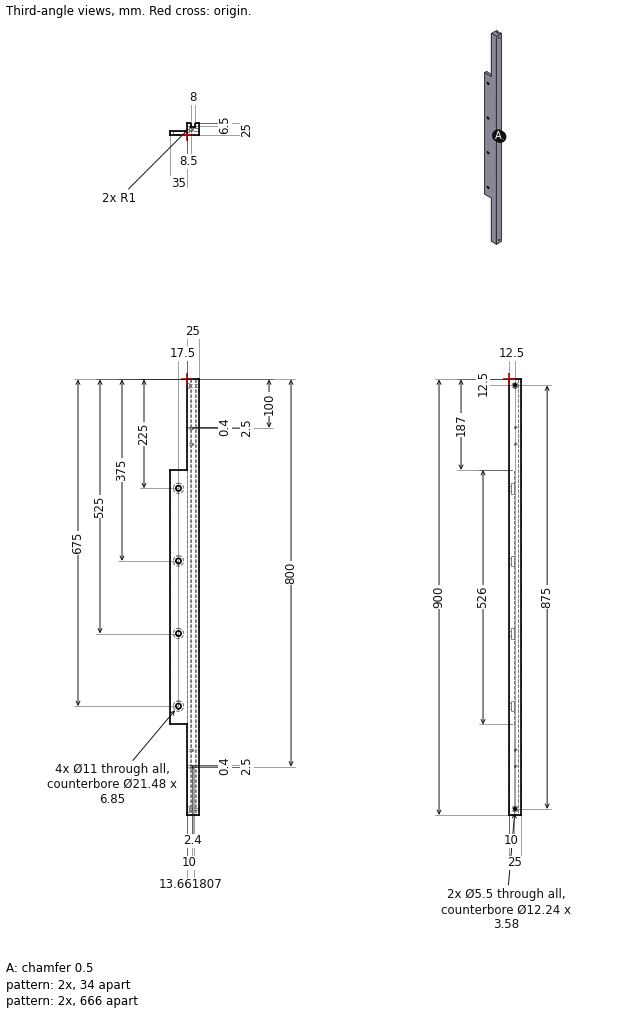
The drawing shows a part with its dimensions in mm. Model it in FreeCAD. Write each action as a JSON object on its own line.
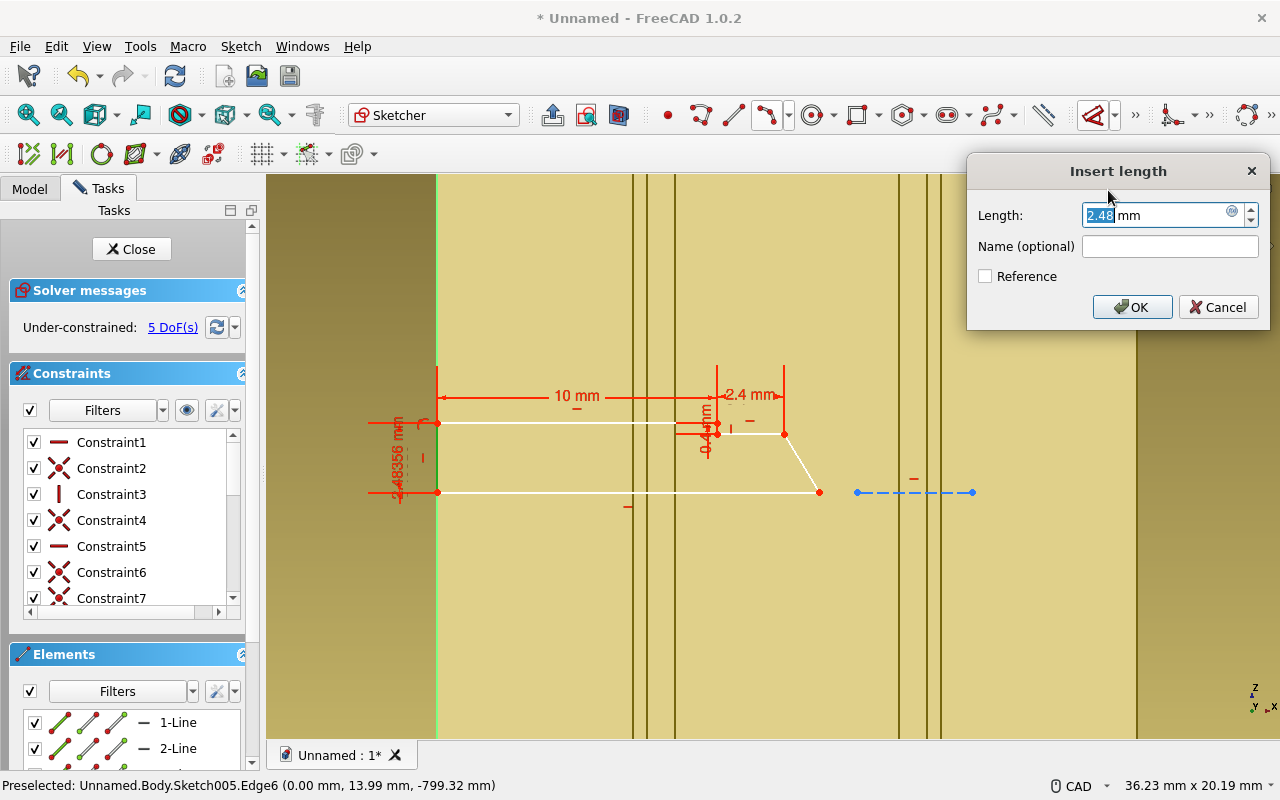
{"action": "type", "text": "2.5"}
{"action": "key", "text": "Return"}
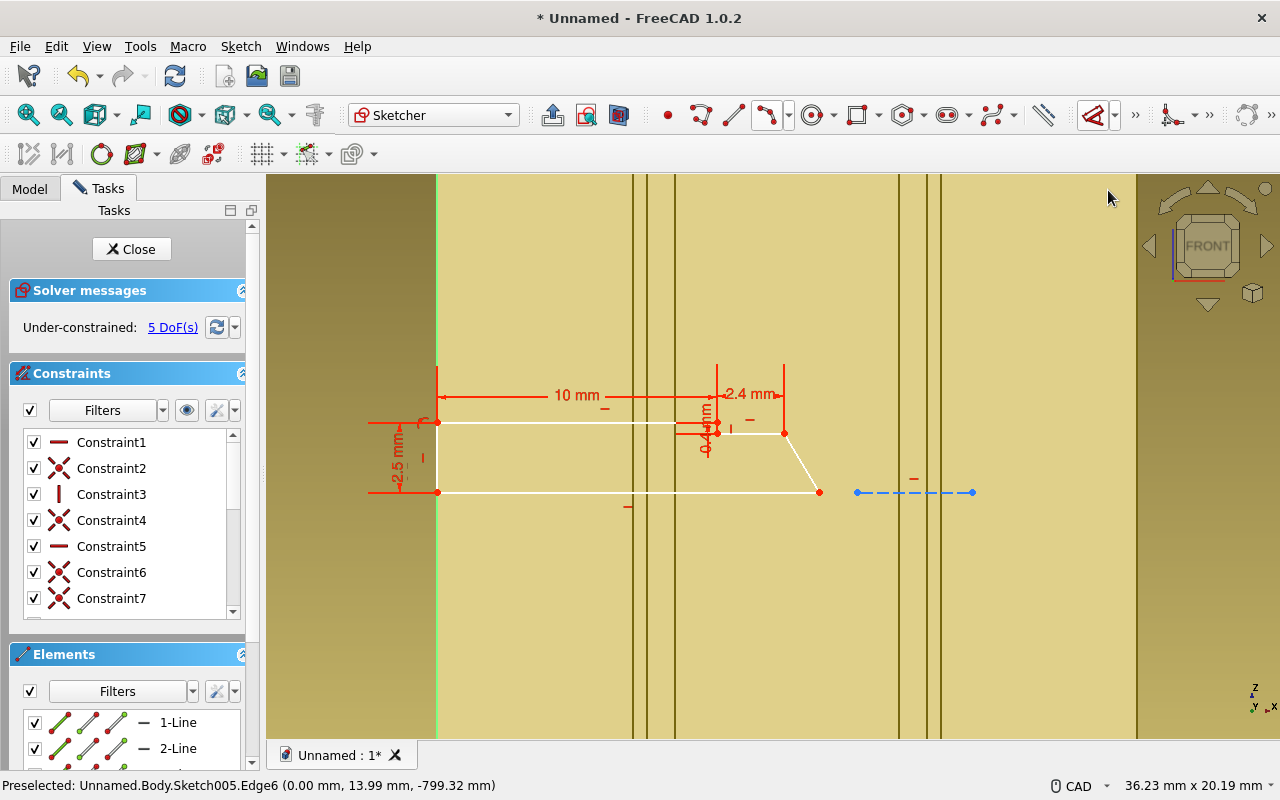
{"action": "left_click", "coordinate": [819, 493]}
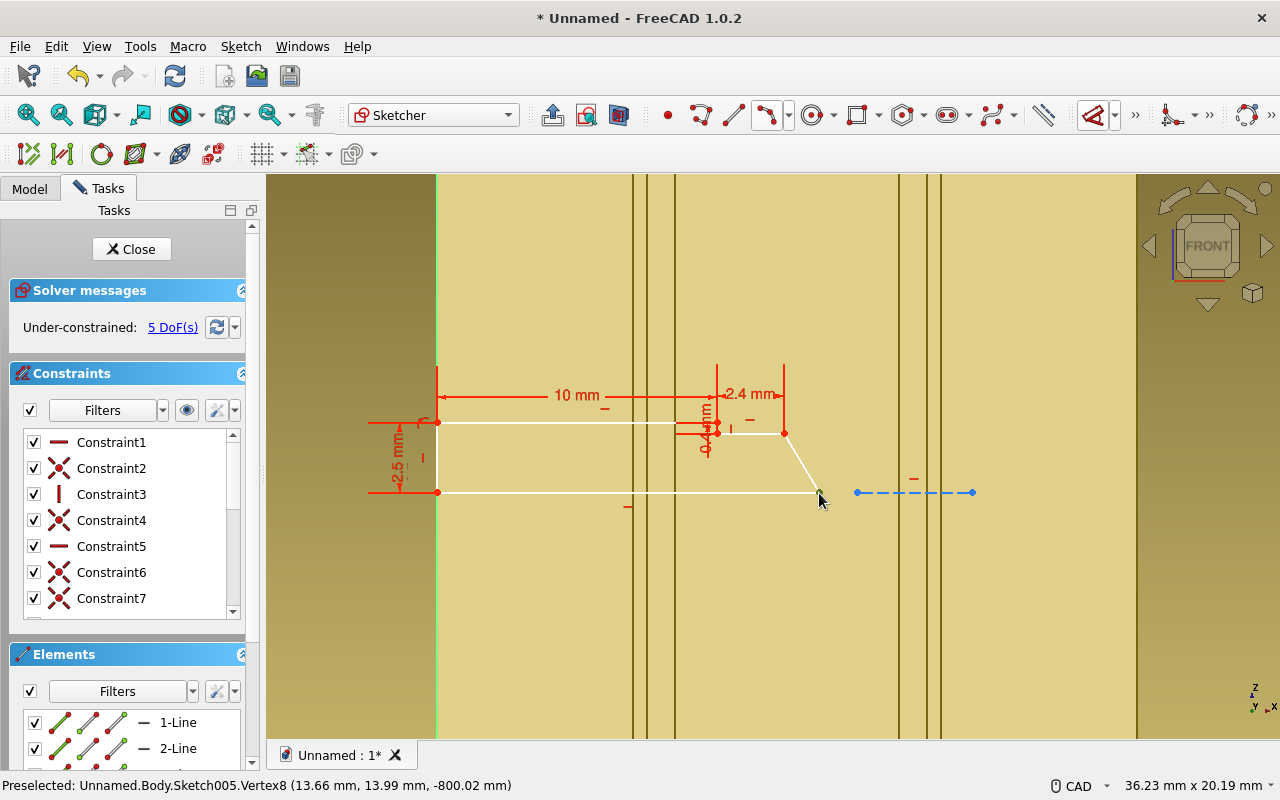
{"action": "left_click", "coordinate": [1114, 116]}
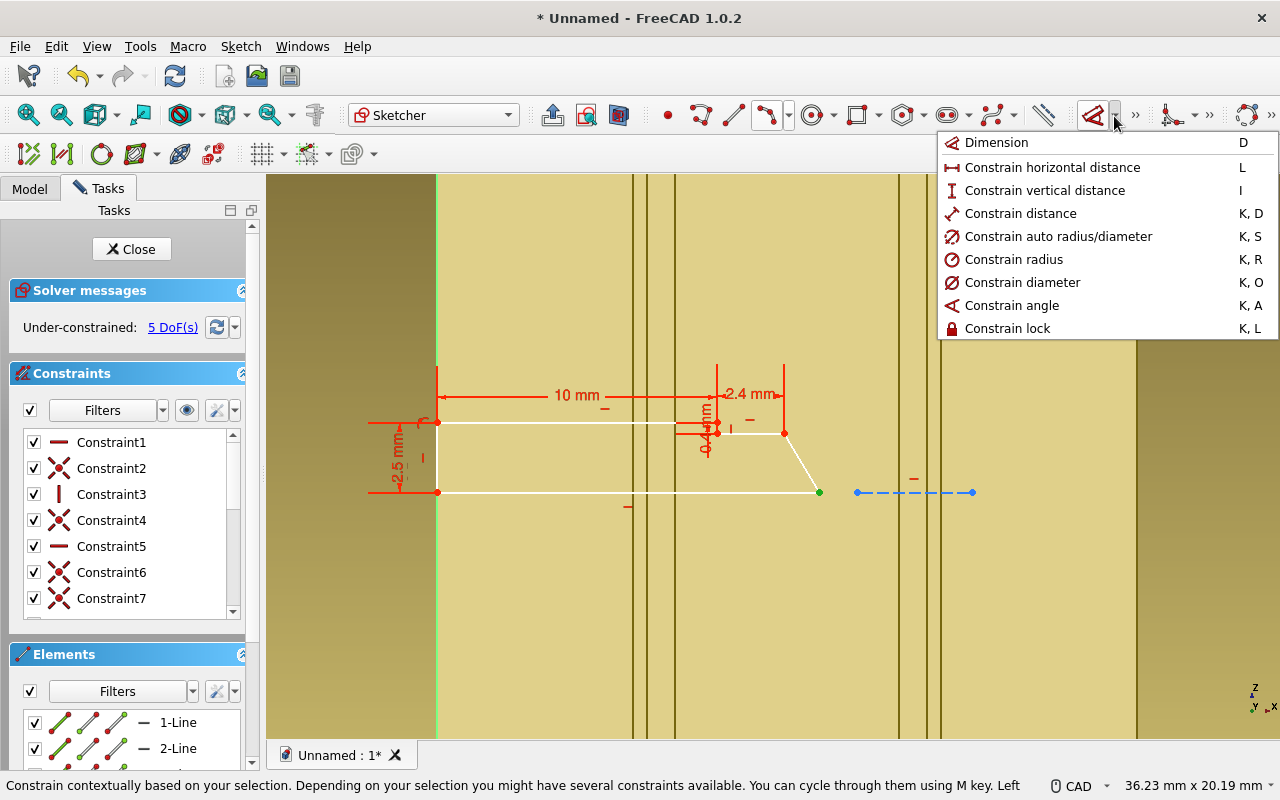
{"action": "left_click", "coordinate": [1108, 190]}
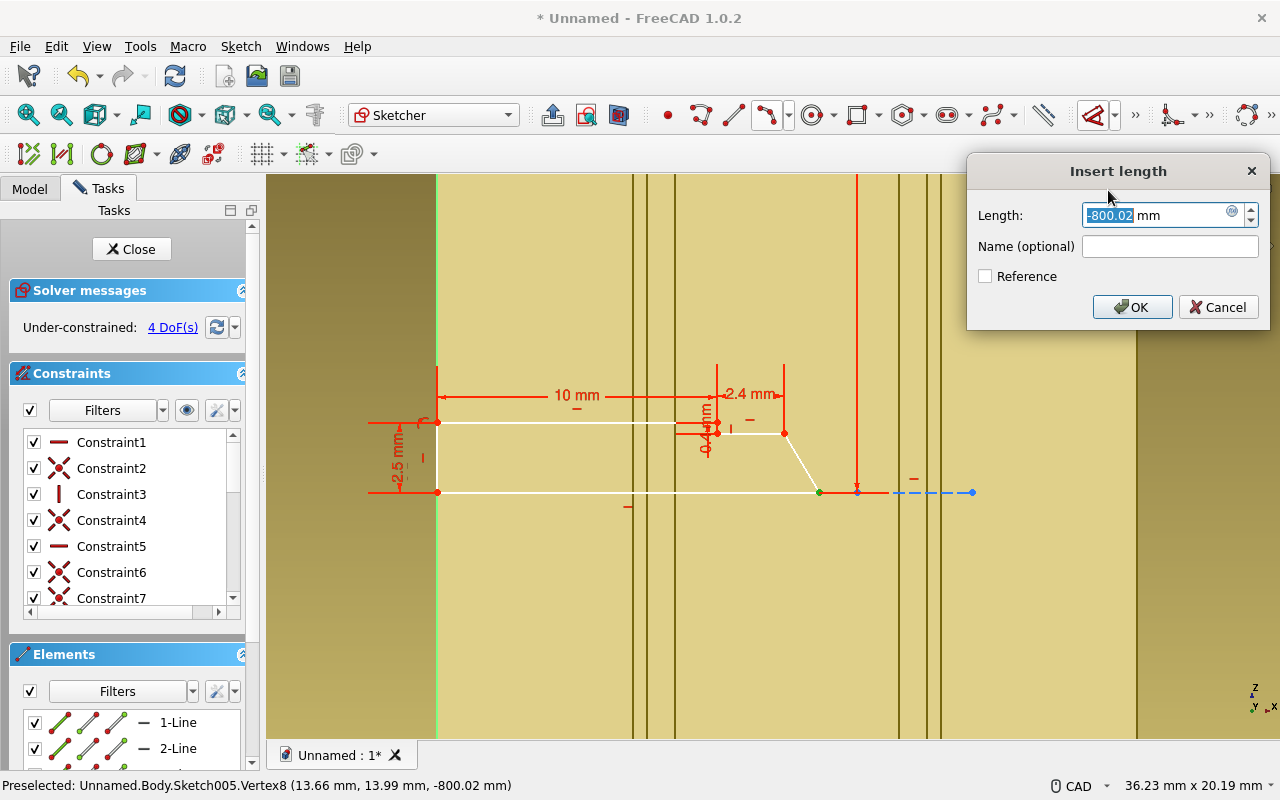
{"action": "type", "text": "-800"}
{"action": "key", "text": "Return"}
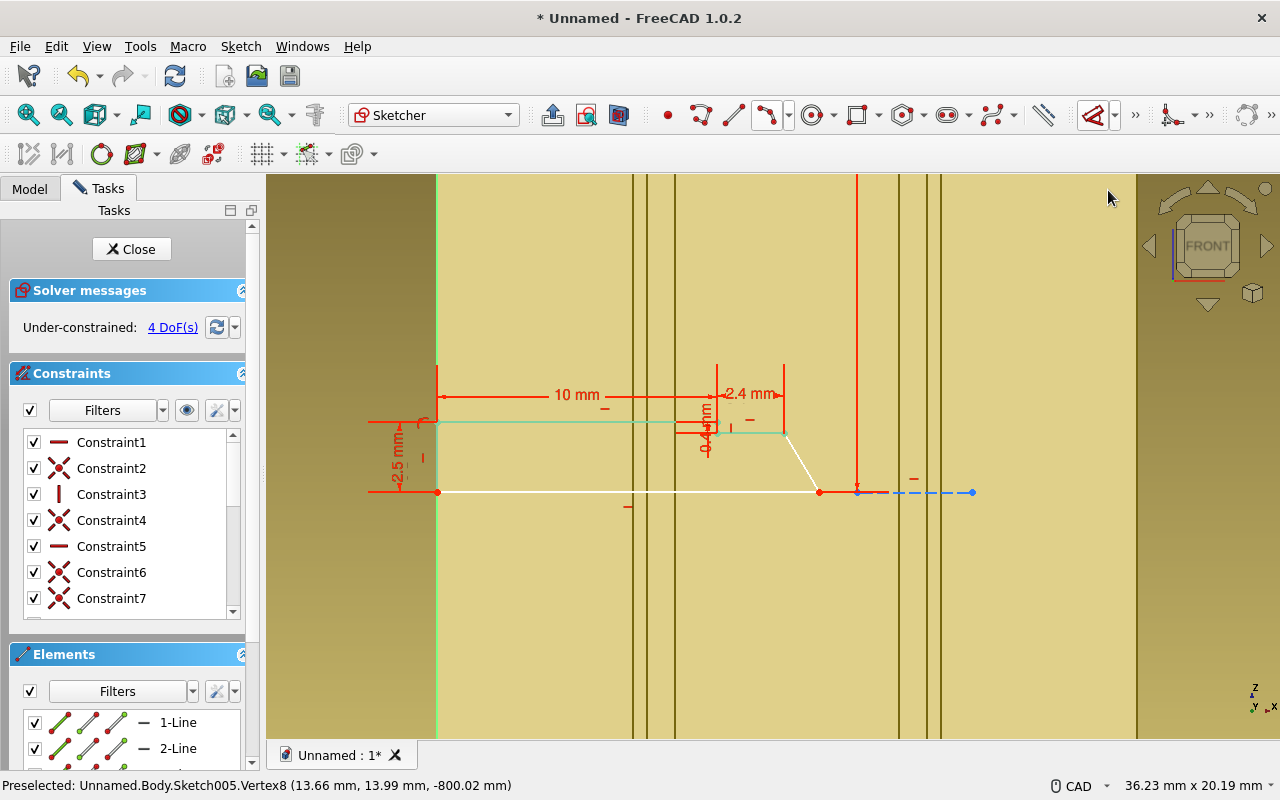
{"action": "left_click", "coordinate": [858, 493]}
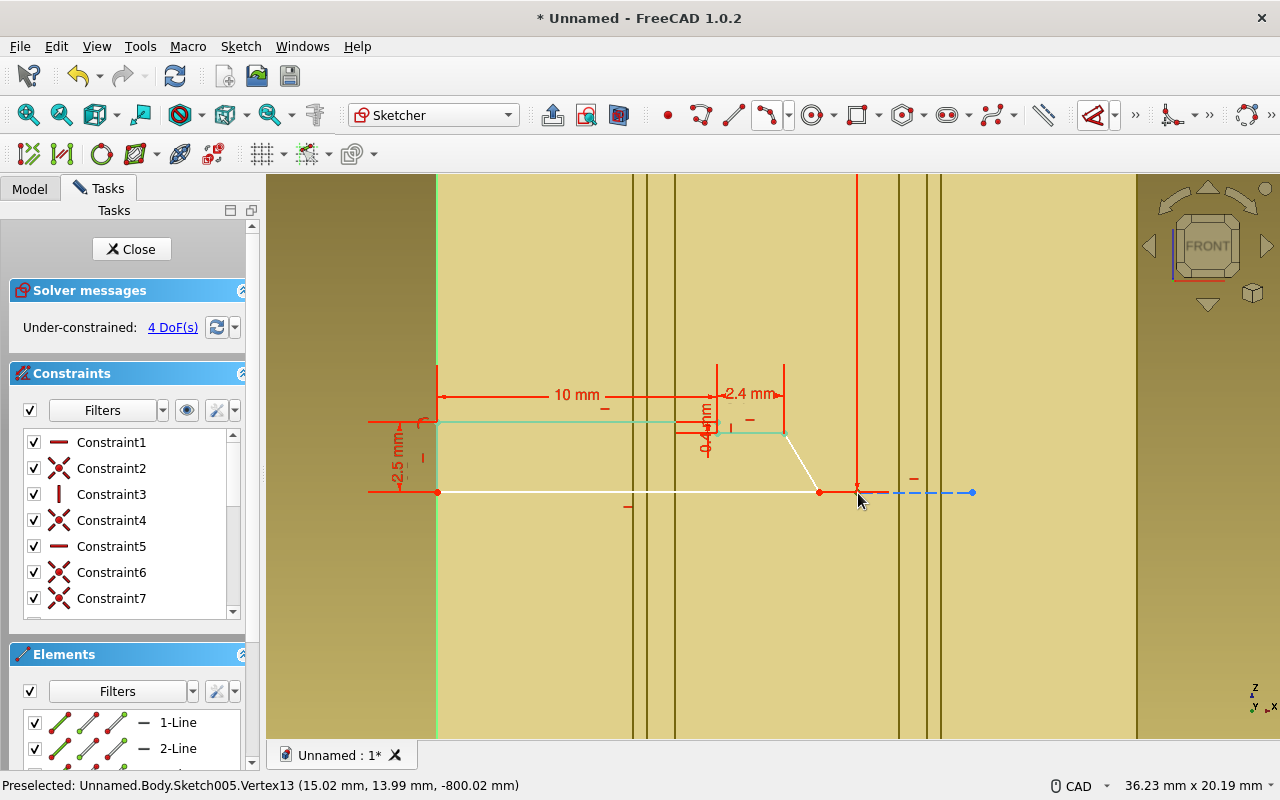
{"action": "key", "text": "i"}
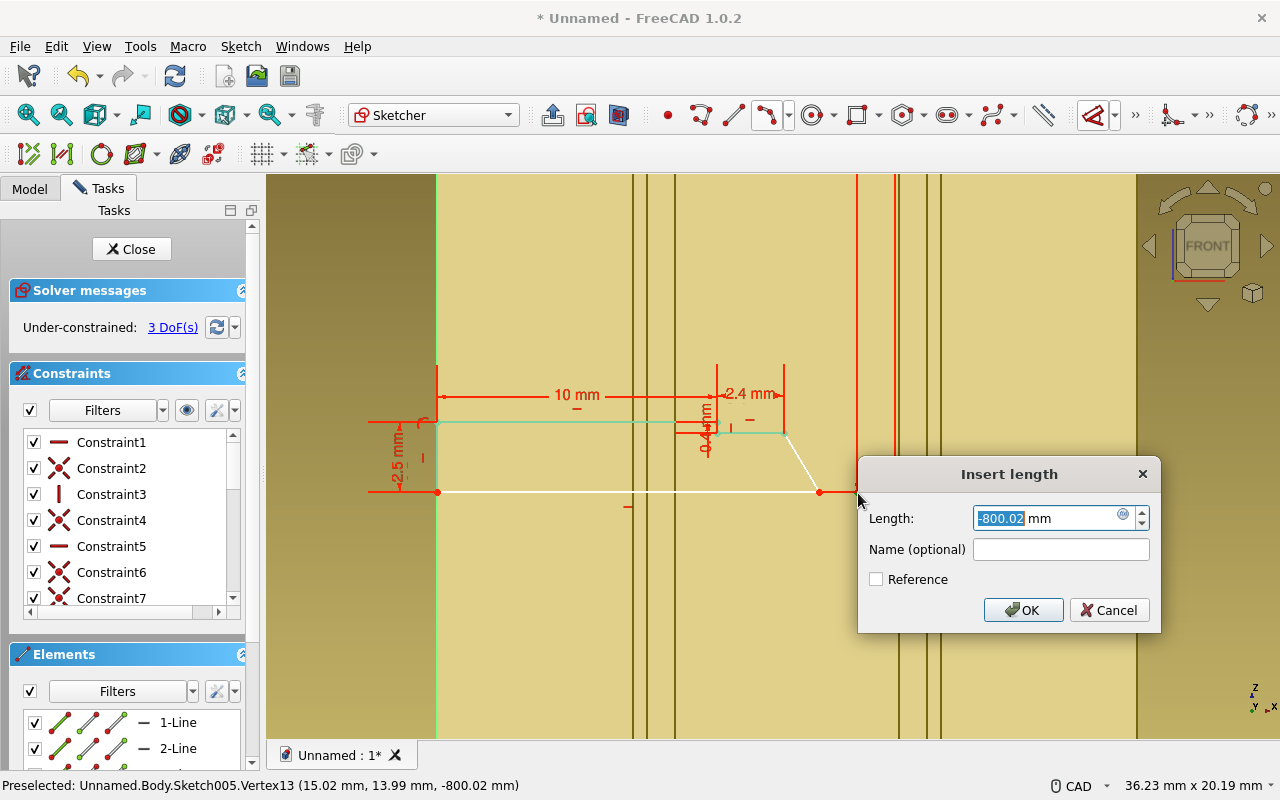
{"action": "type", "text": "-800"}
{"action": "key", "text": "Return"}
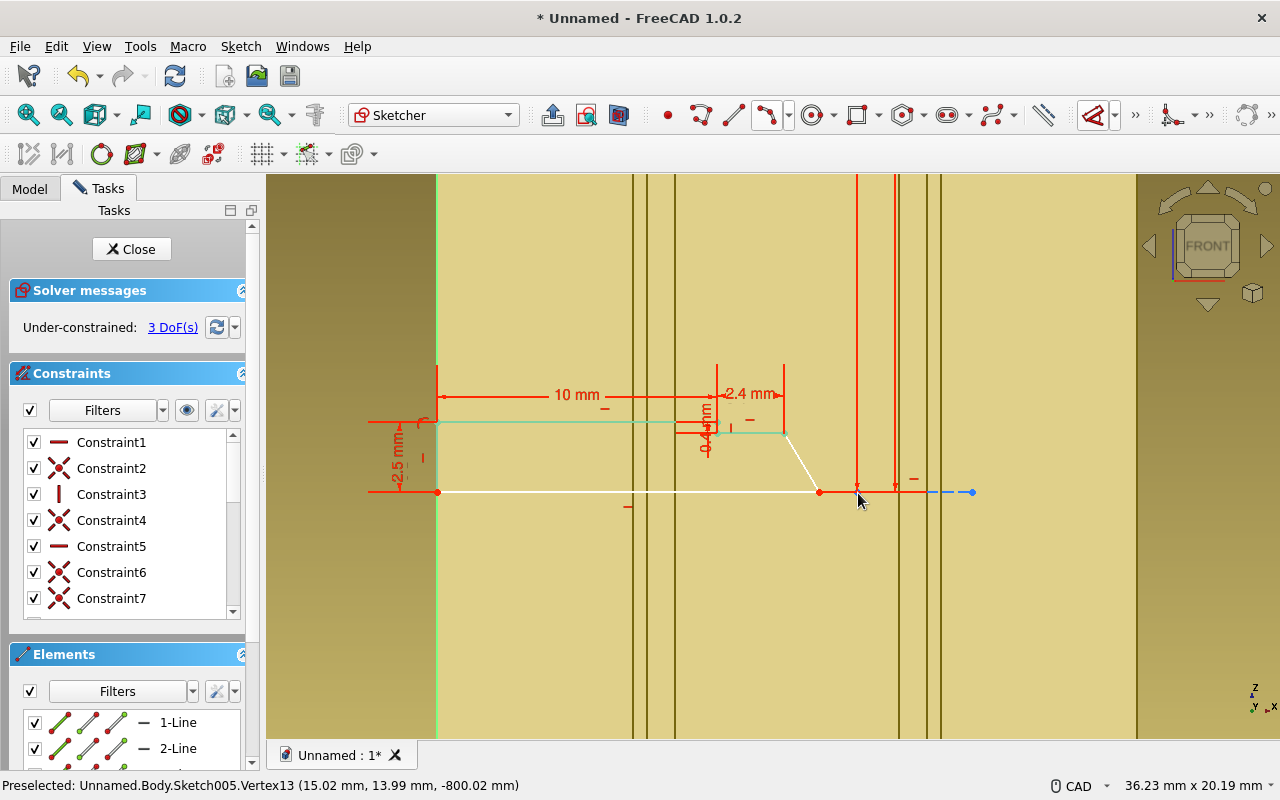
{"action": "left_click", "coordinate": [705, 492]}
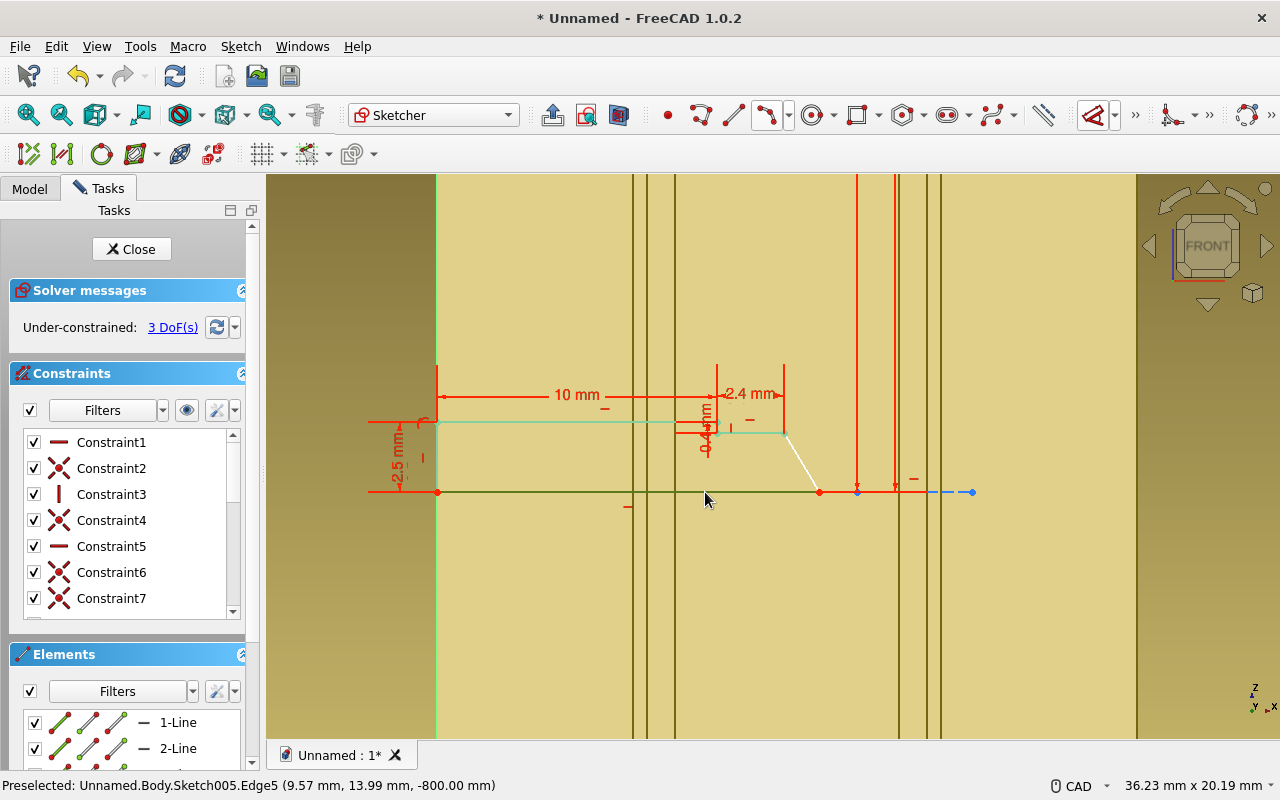
{"action": "key", "text": "l"}